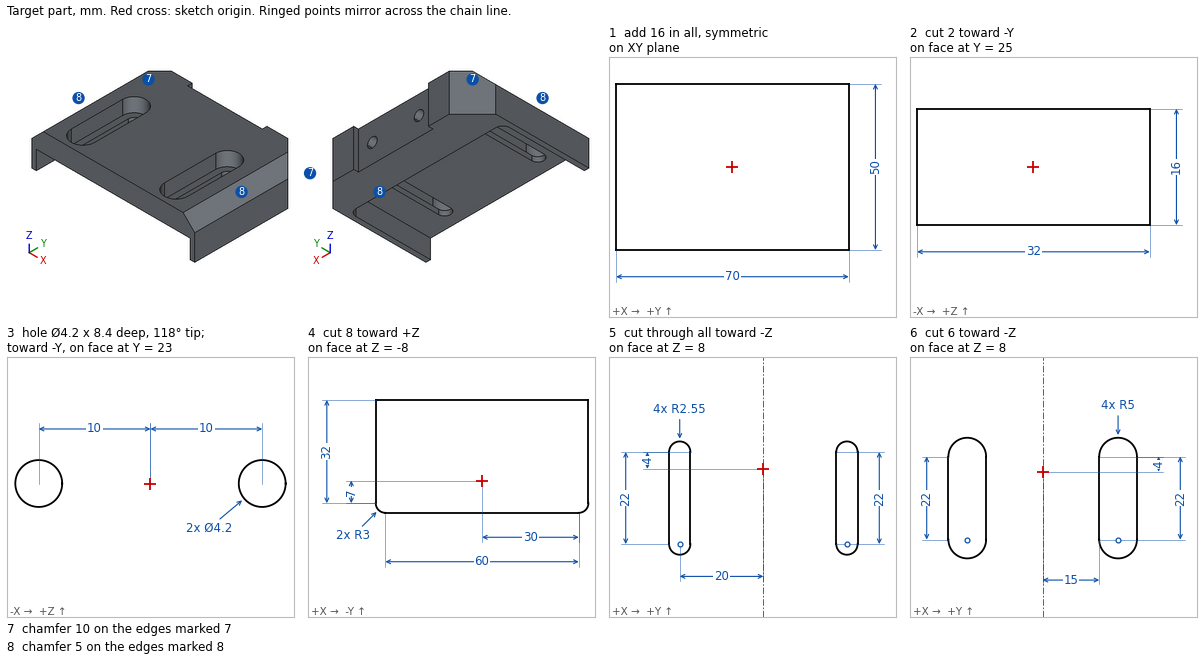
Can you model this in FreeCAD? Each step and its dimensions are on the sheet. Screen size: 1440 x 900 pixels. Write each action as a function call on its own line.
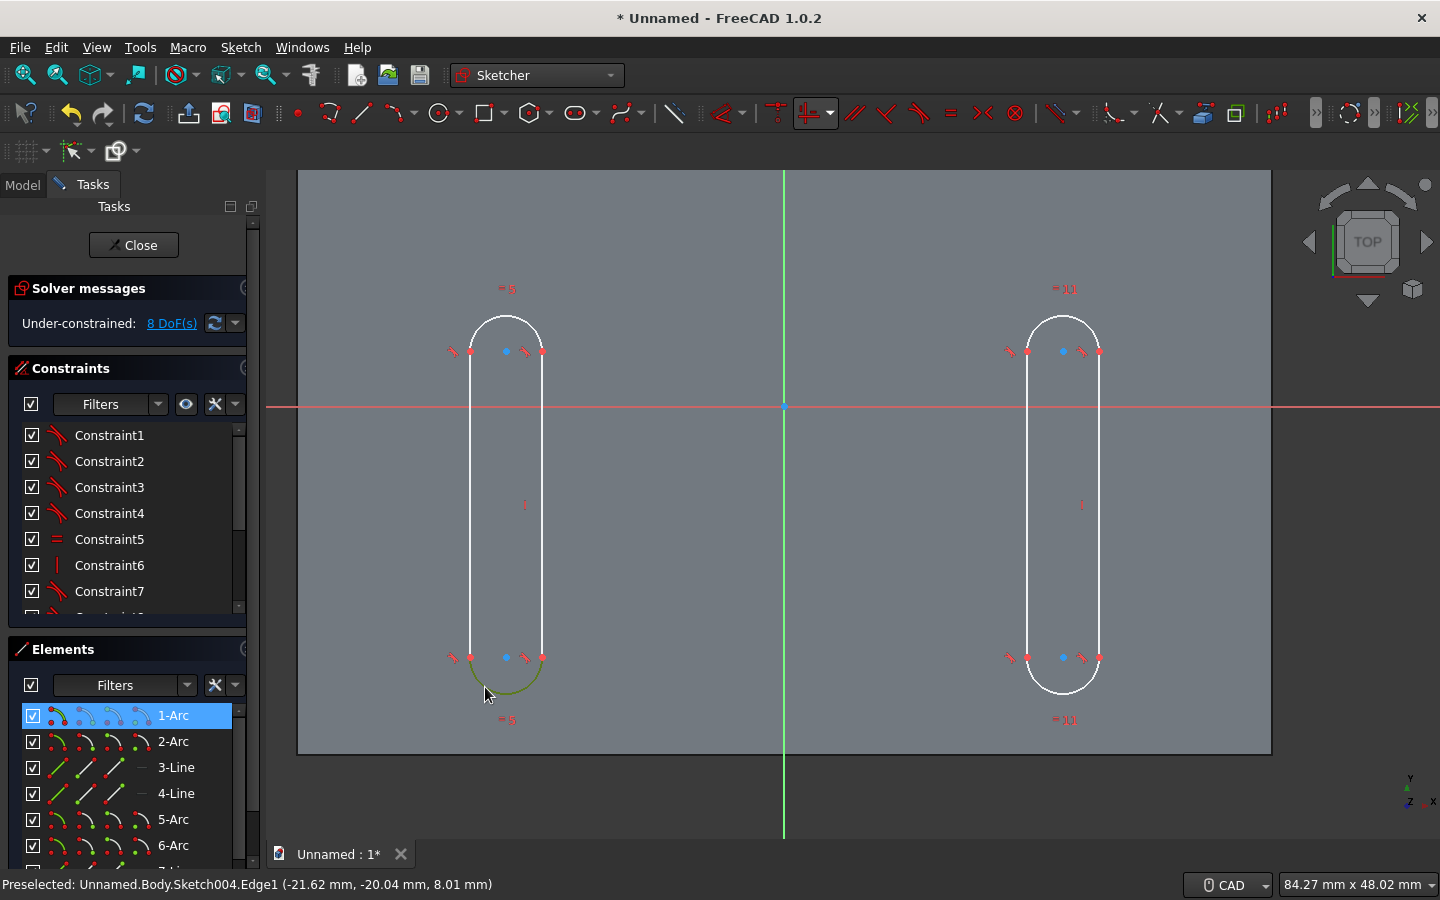
click(1042, 687)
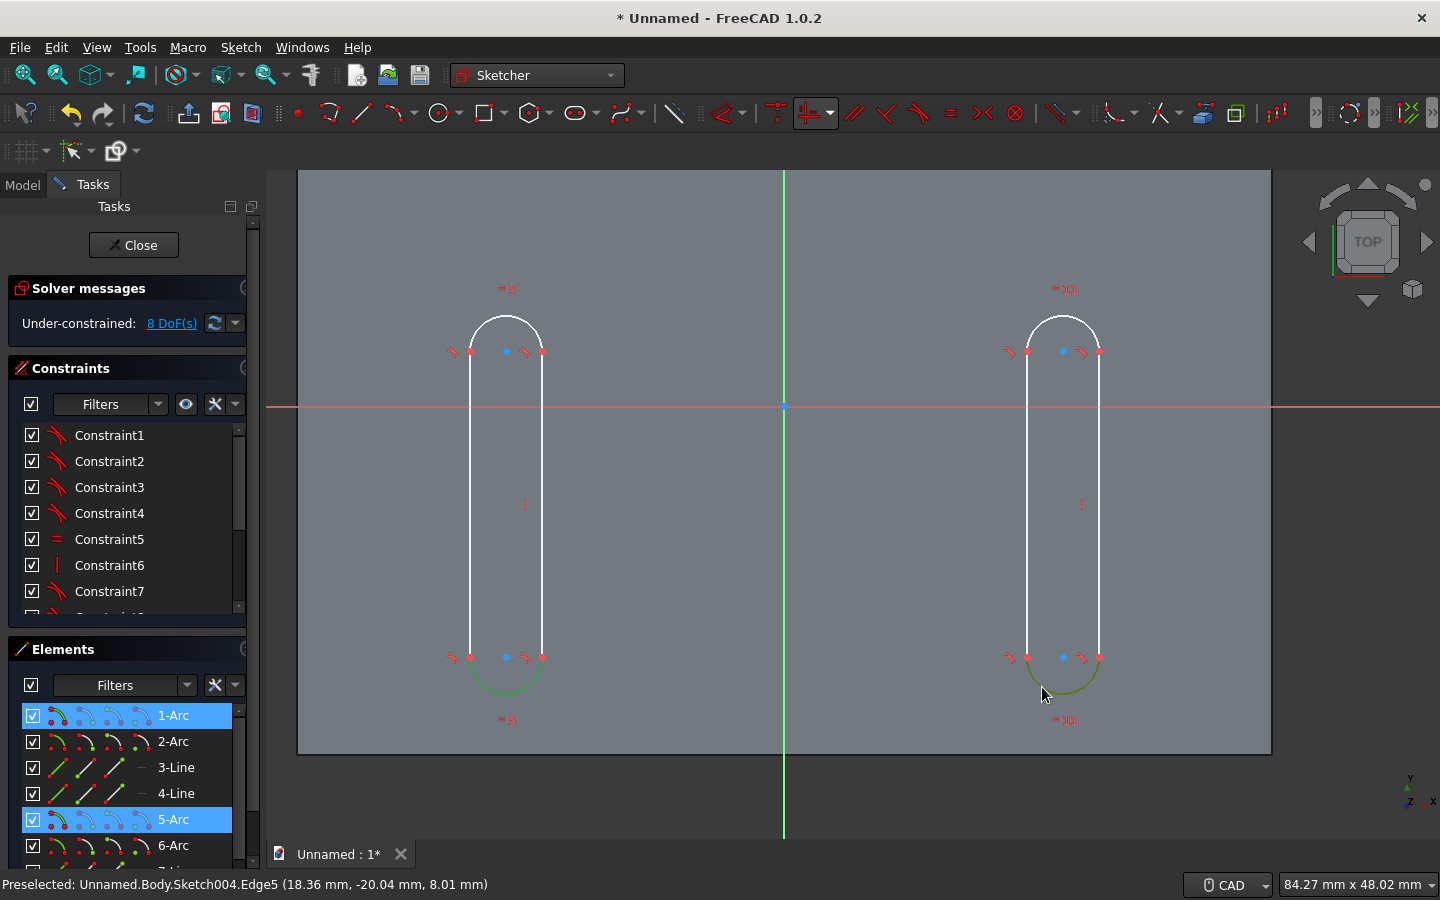
click(952, 114)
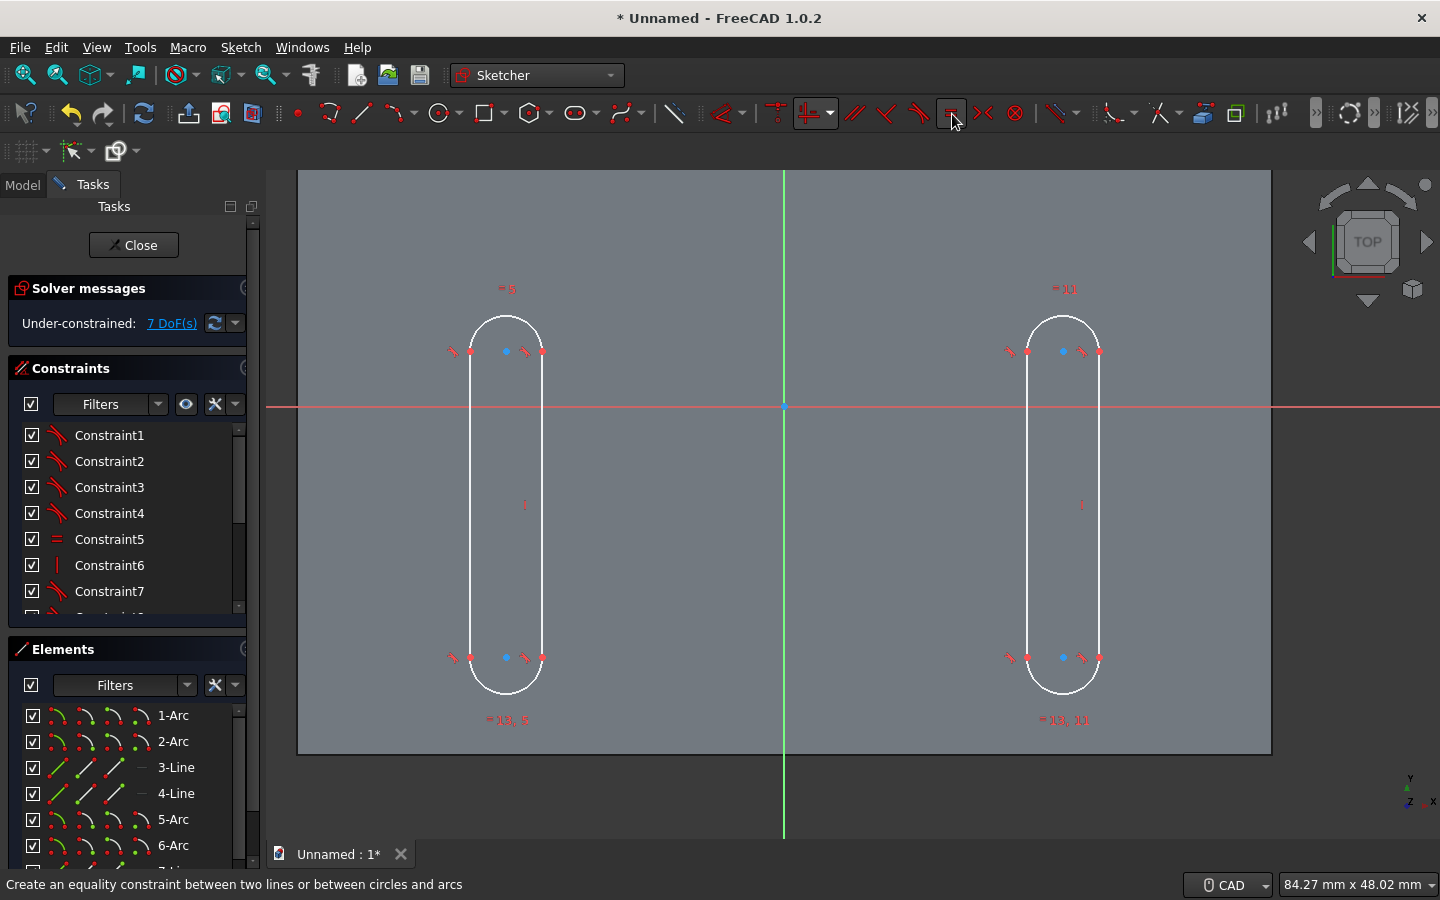
click(506, 658)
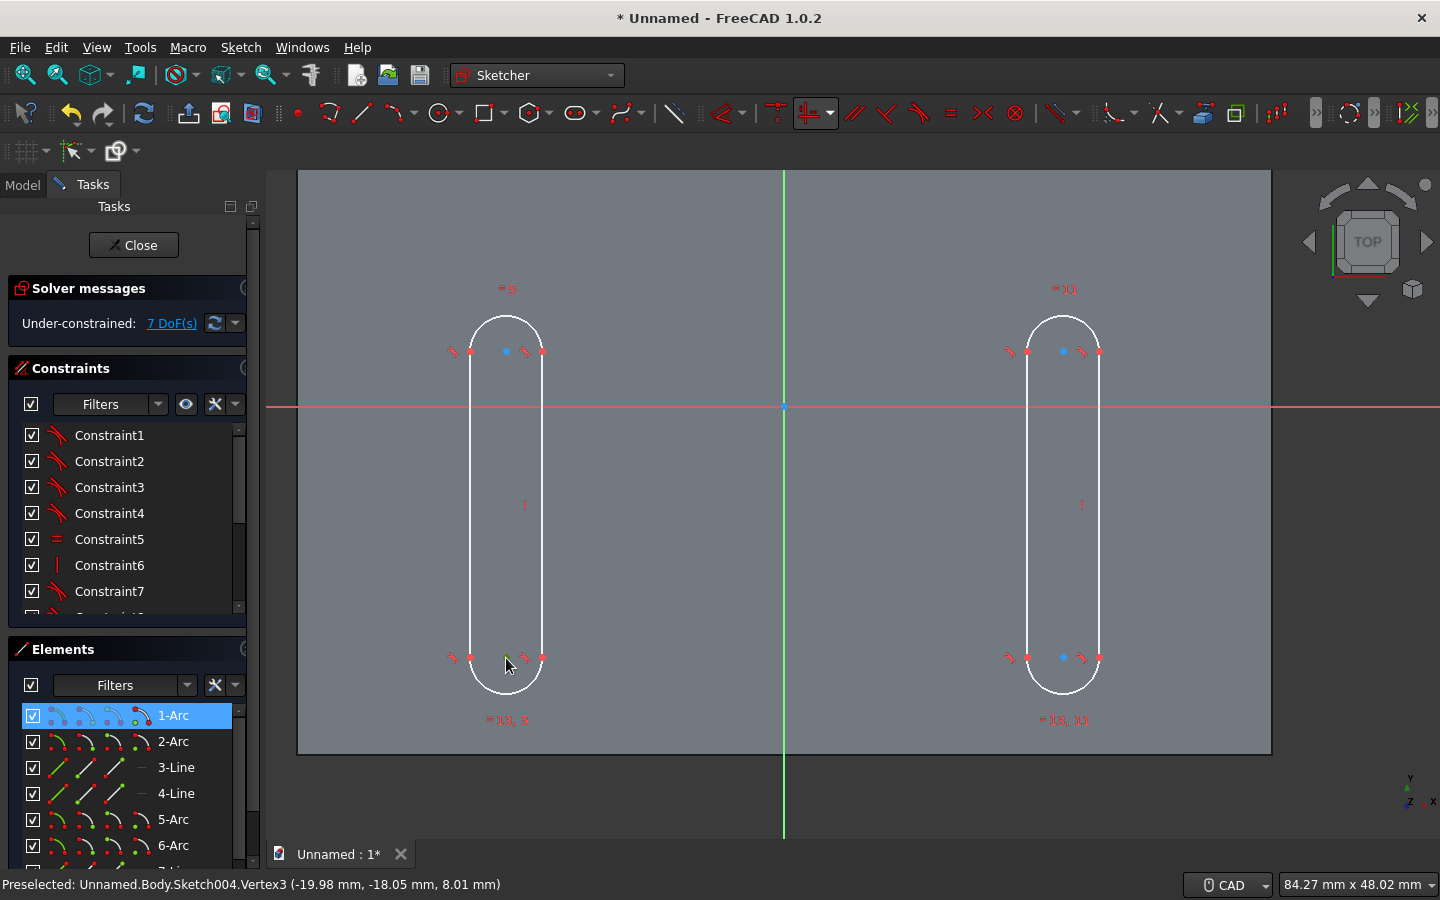
click(1063, 658)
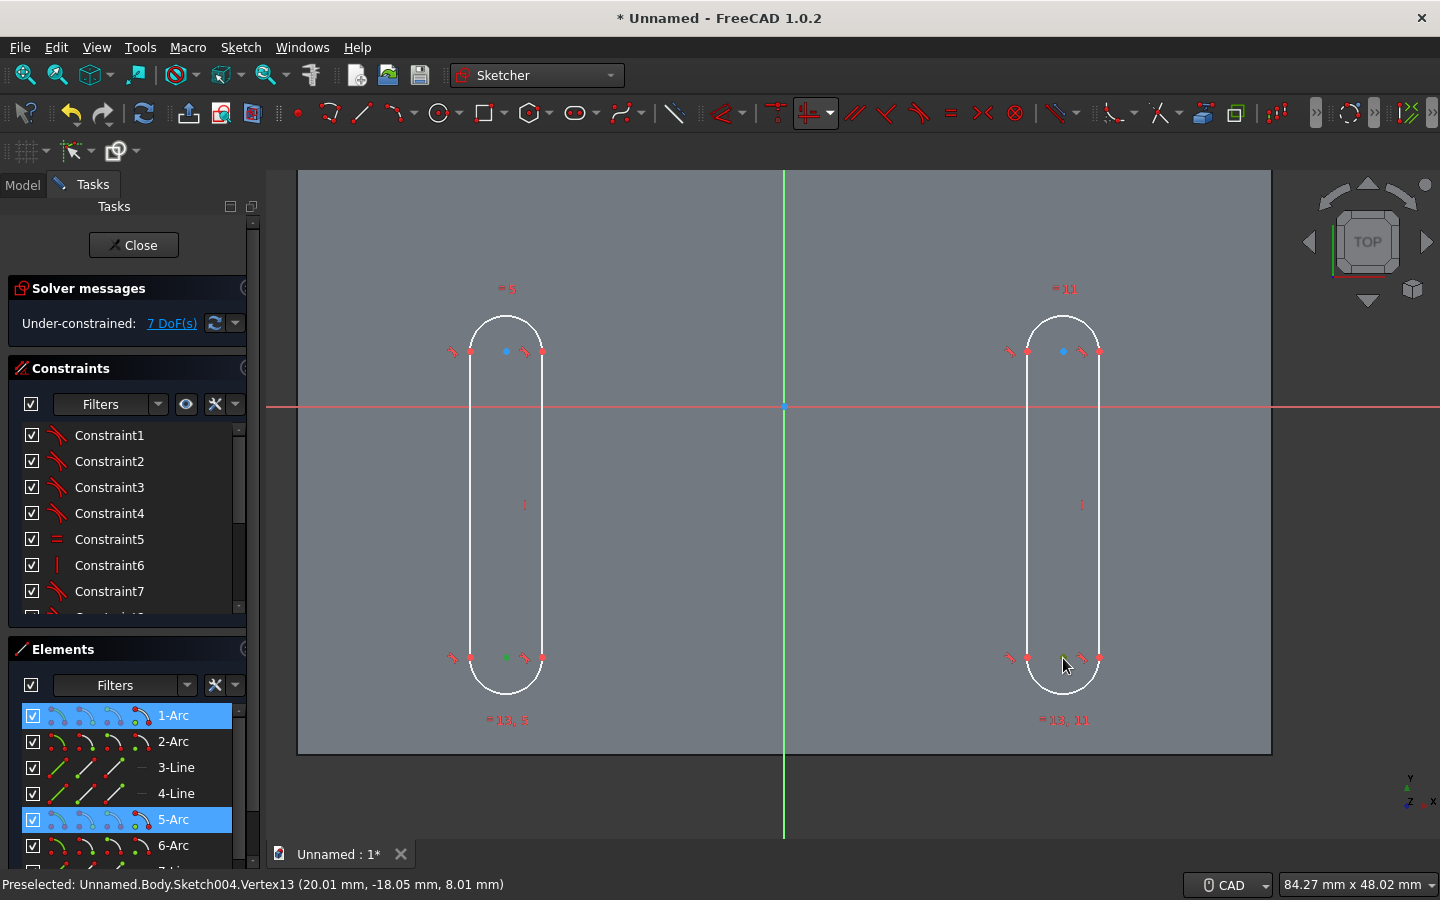
click(784, 767)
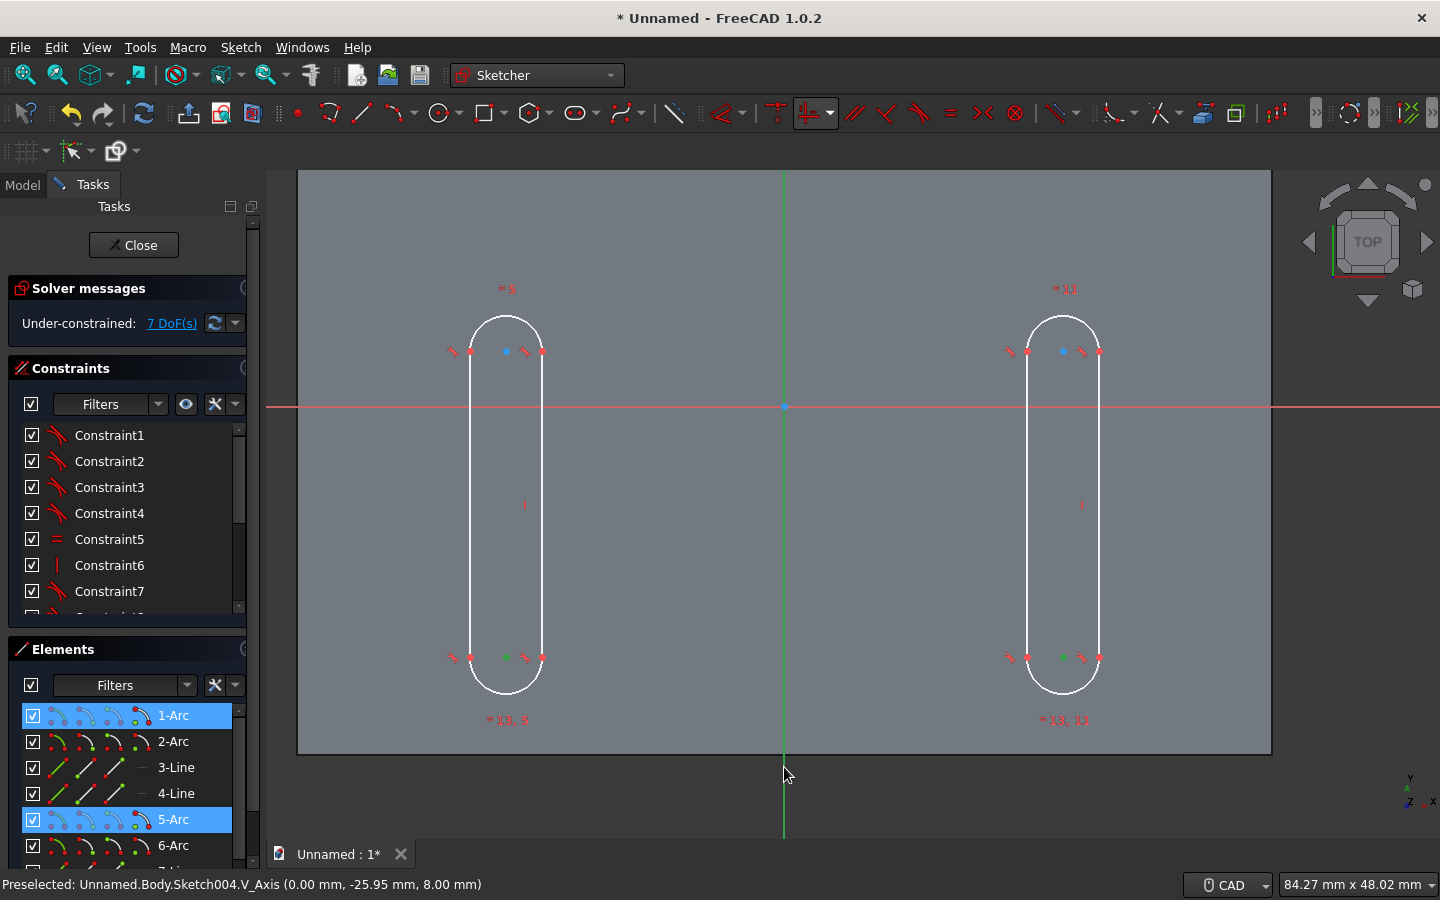
click(984, 114)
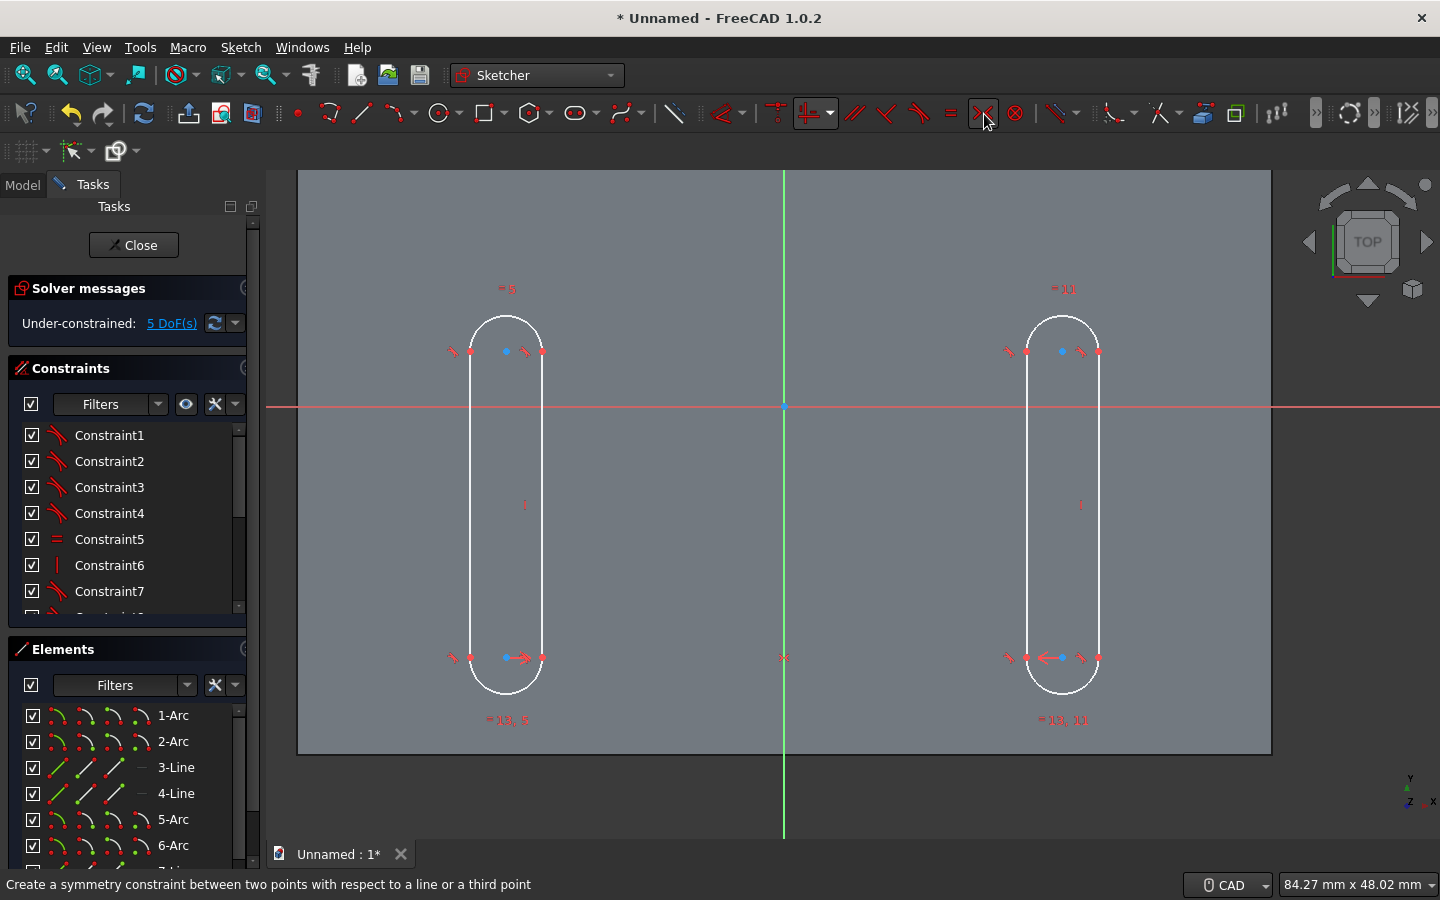
click(722, 114)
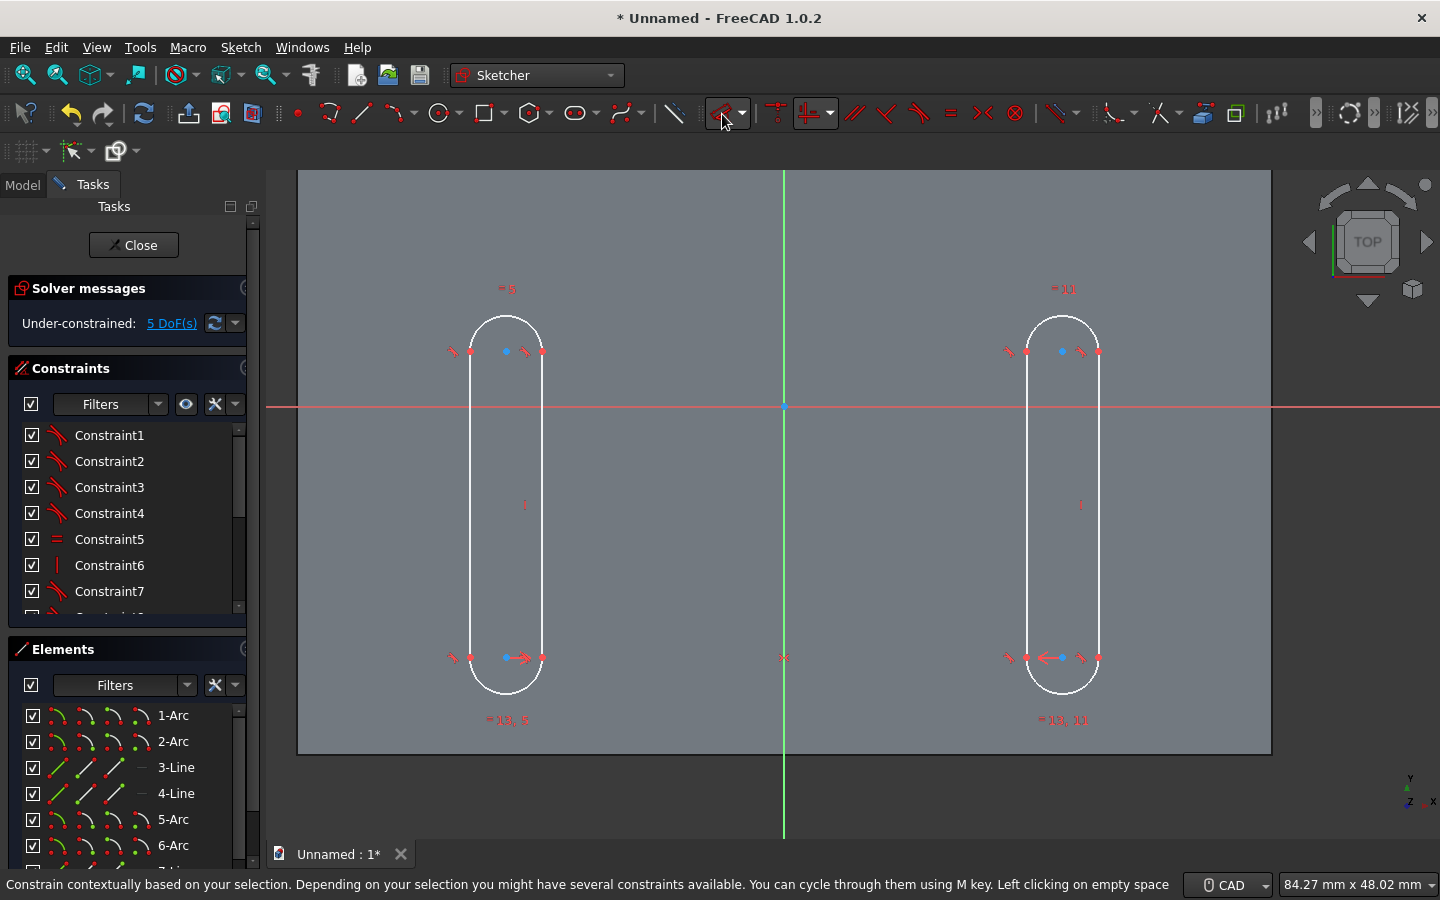
click(485, 687)
click(466, 713)